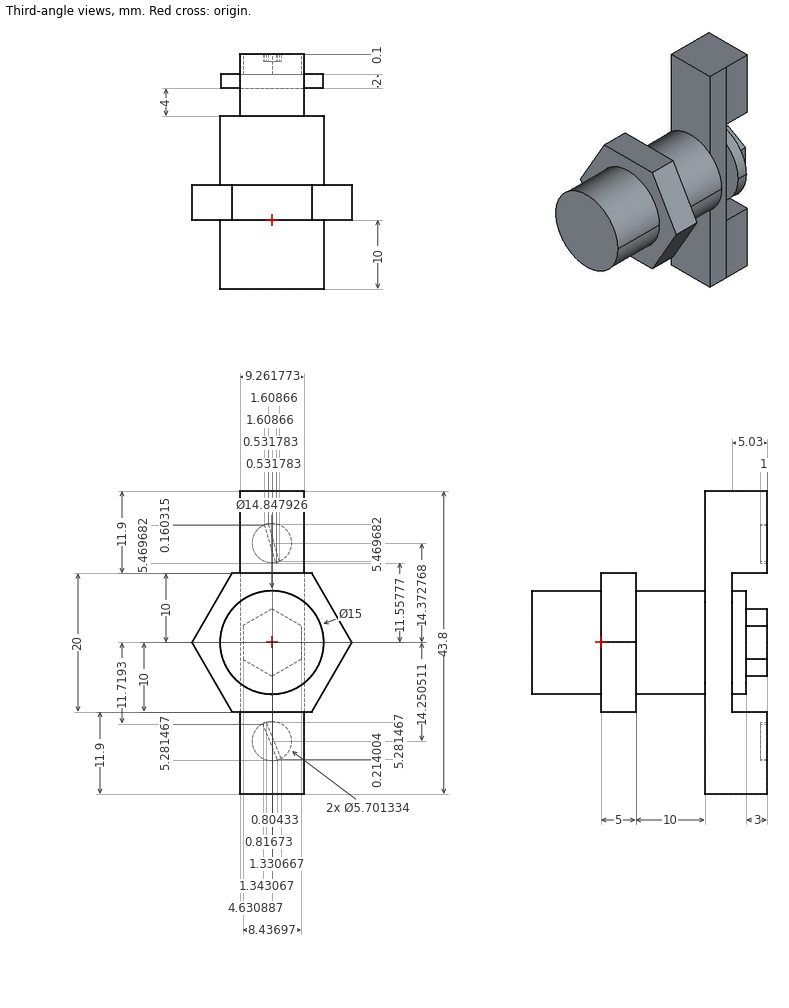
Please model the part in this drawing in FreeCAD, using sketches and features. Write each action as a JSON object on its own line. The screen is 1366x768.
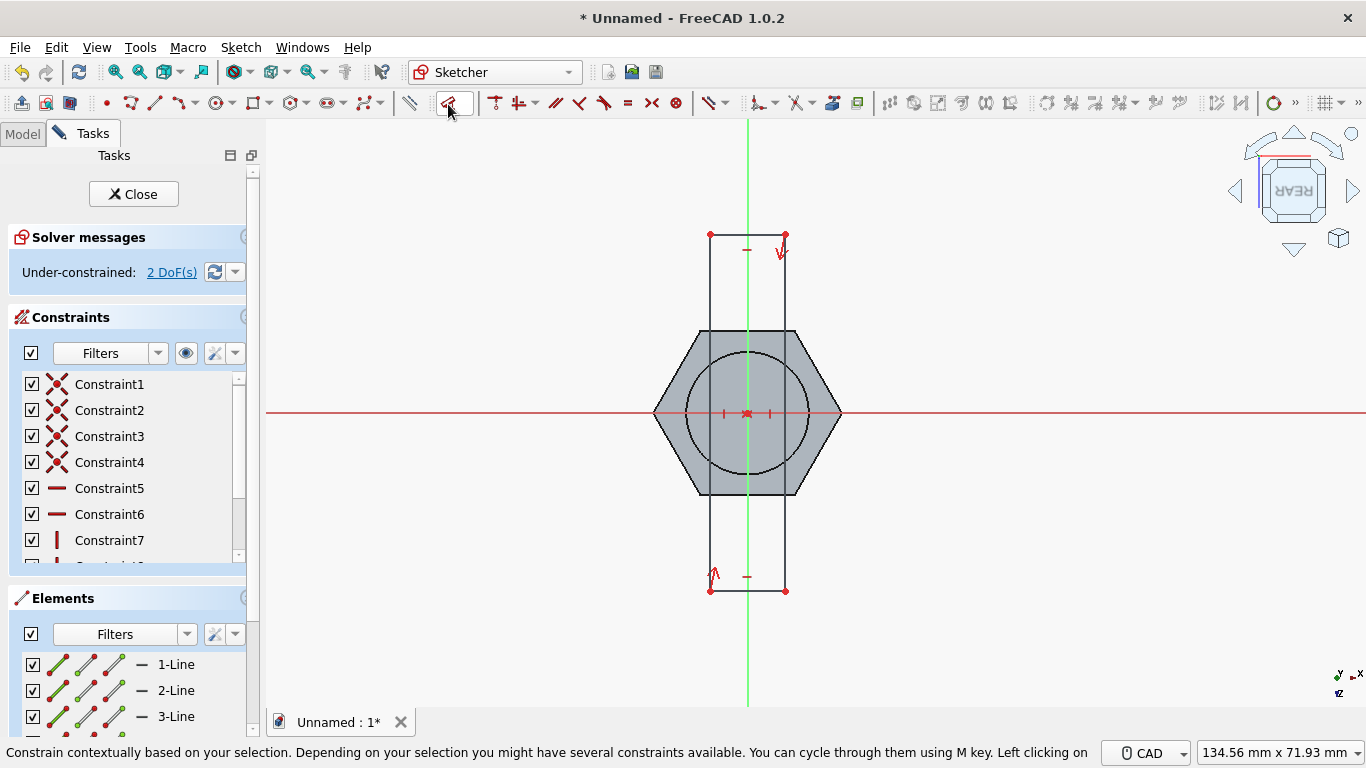
{"action": "left_click", "coordinate": [785, 485]}
{"action": "left_click", "coordinate": [819, 331]}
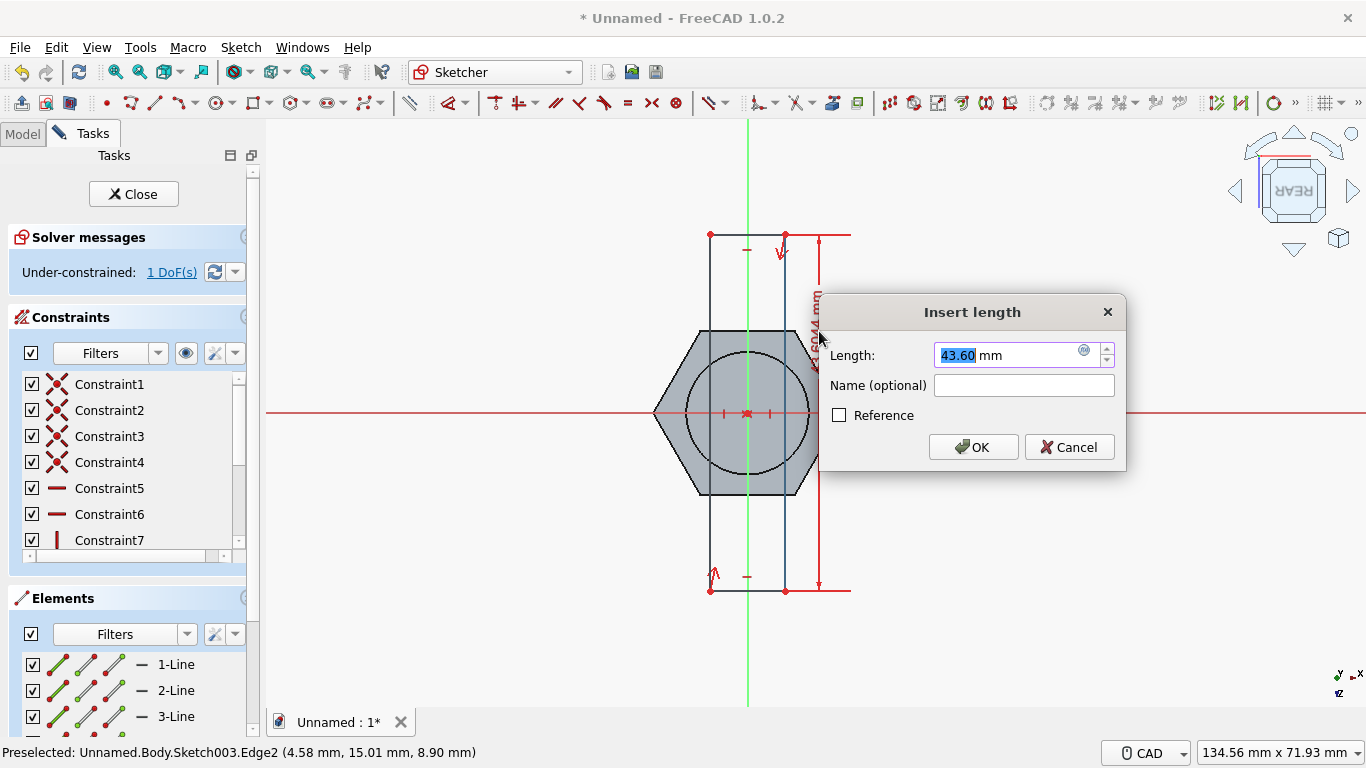
{"action": "type", "text": "43.8"}
{"action": "key", "text": "Return"}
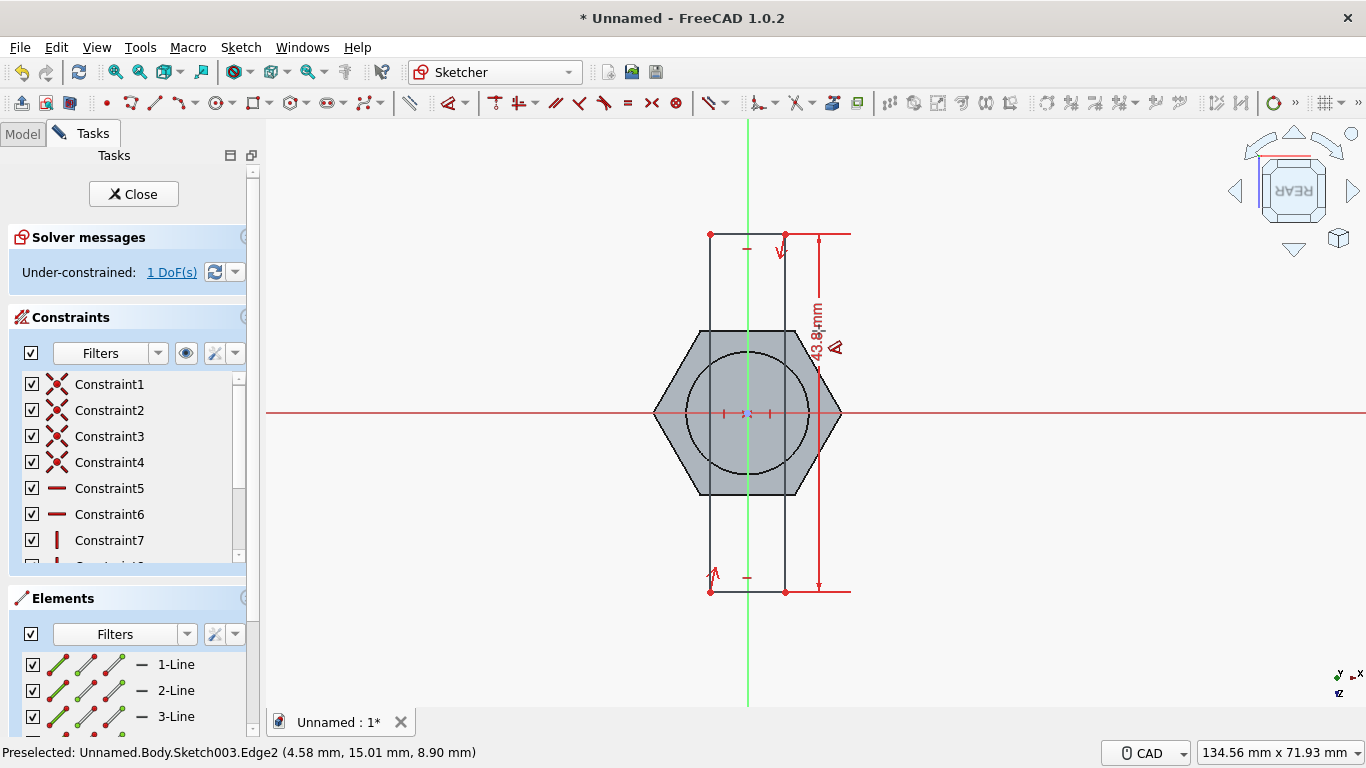
{"action": "left_click", "coordinate": [733, 592]}
{"action": "left_click", "coordinate": [730, 626]}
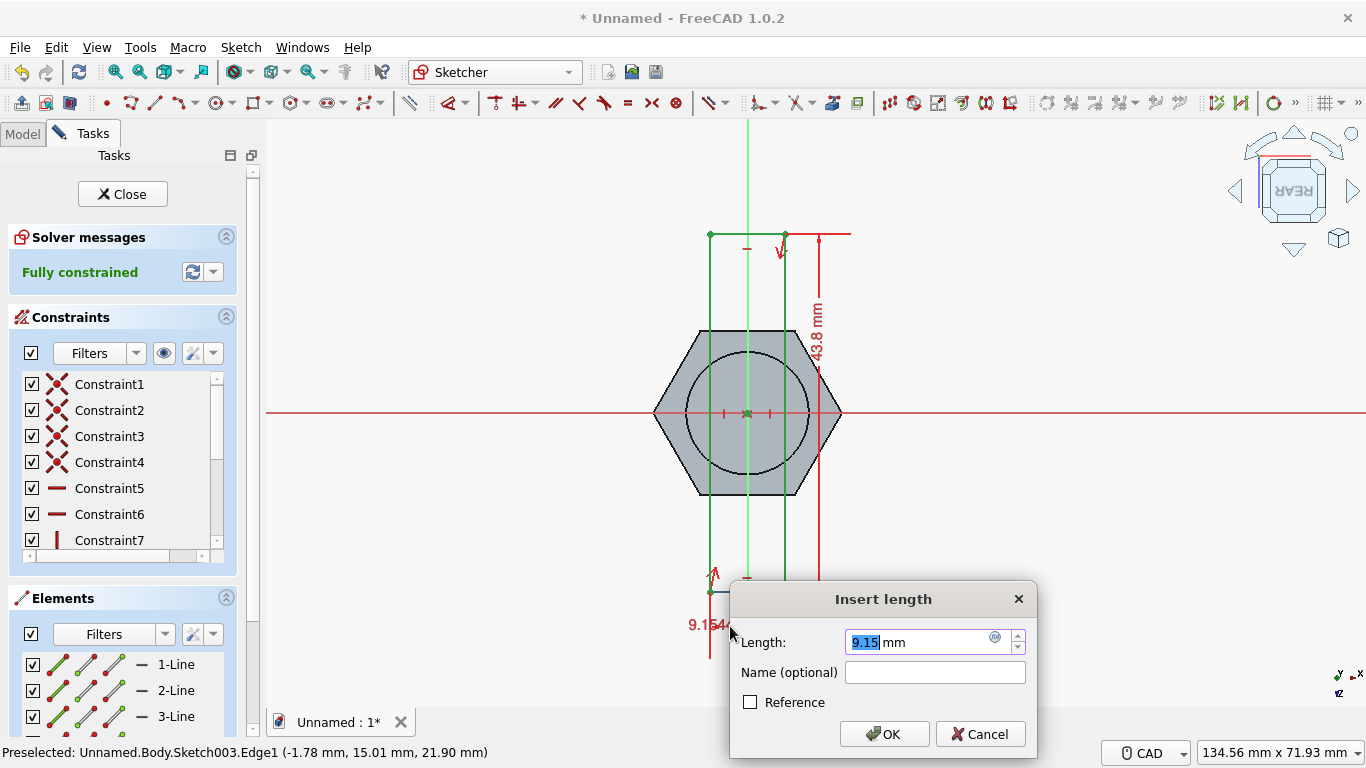
{"action": "type", "text": "9.261773"}
{"action": "key", "text": "Return"}
{"action": "key", "text": "Escape"}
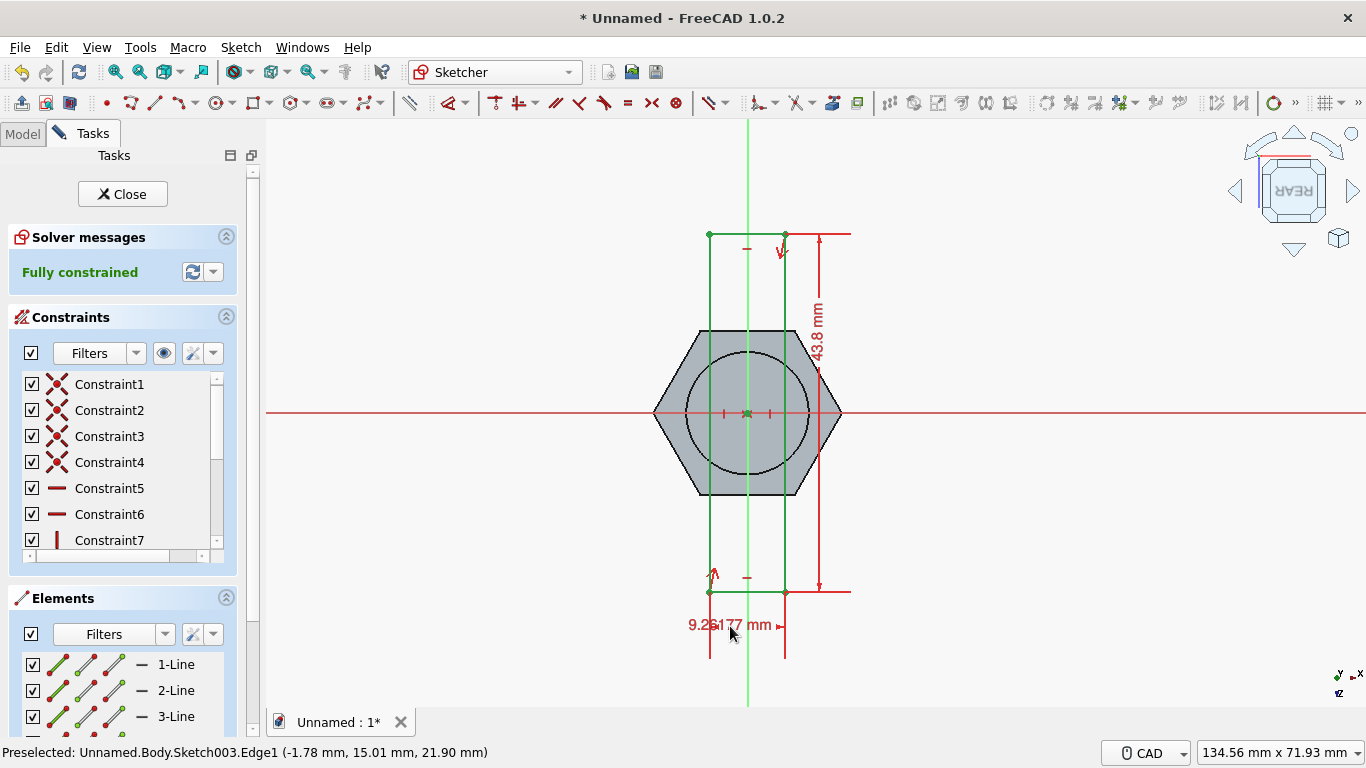
{"action": "left_click", "coordinate": [123, 194]}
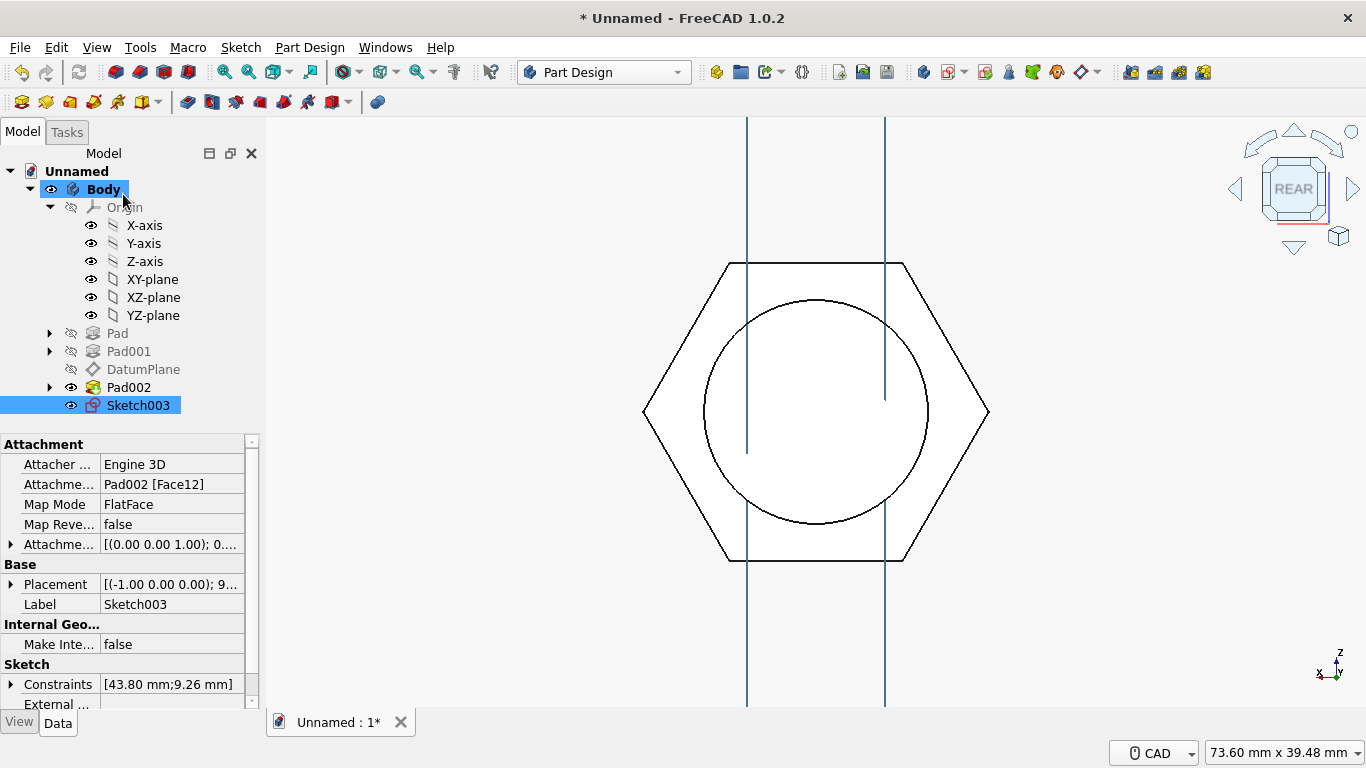
{"action": "left_click", "coordinate": [22, 102]}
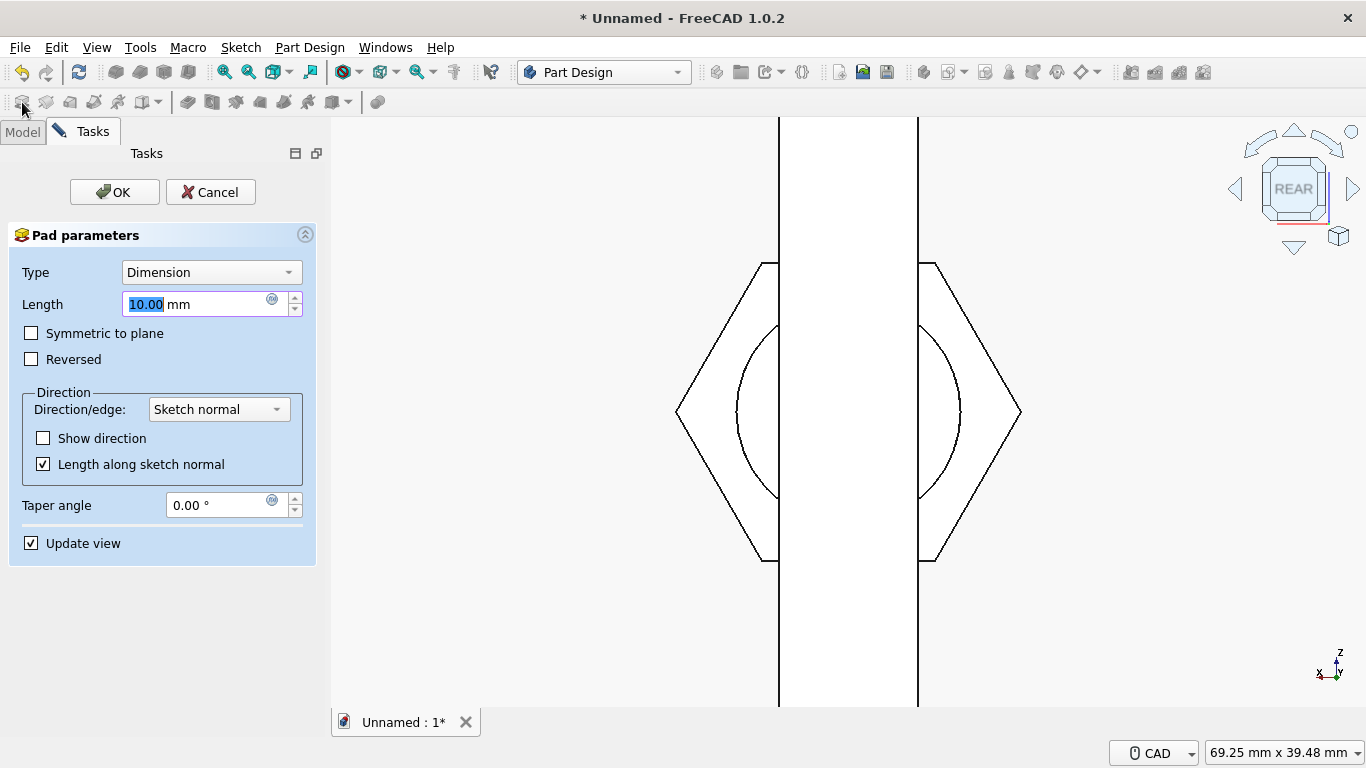
{"action": "type", "text": "4"}
{"action": "key", "text": "Tab"}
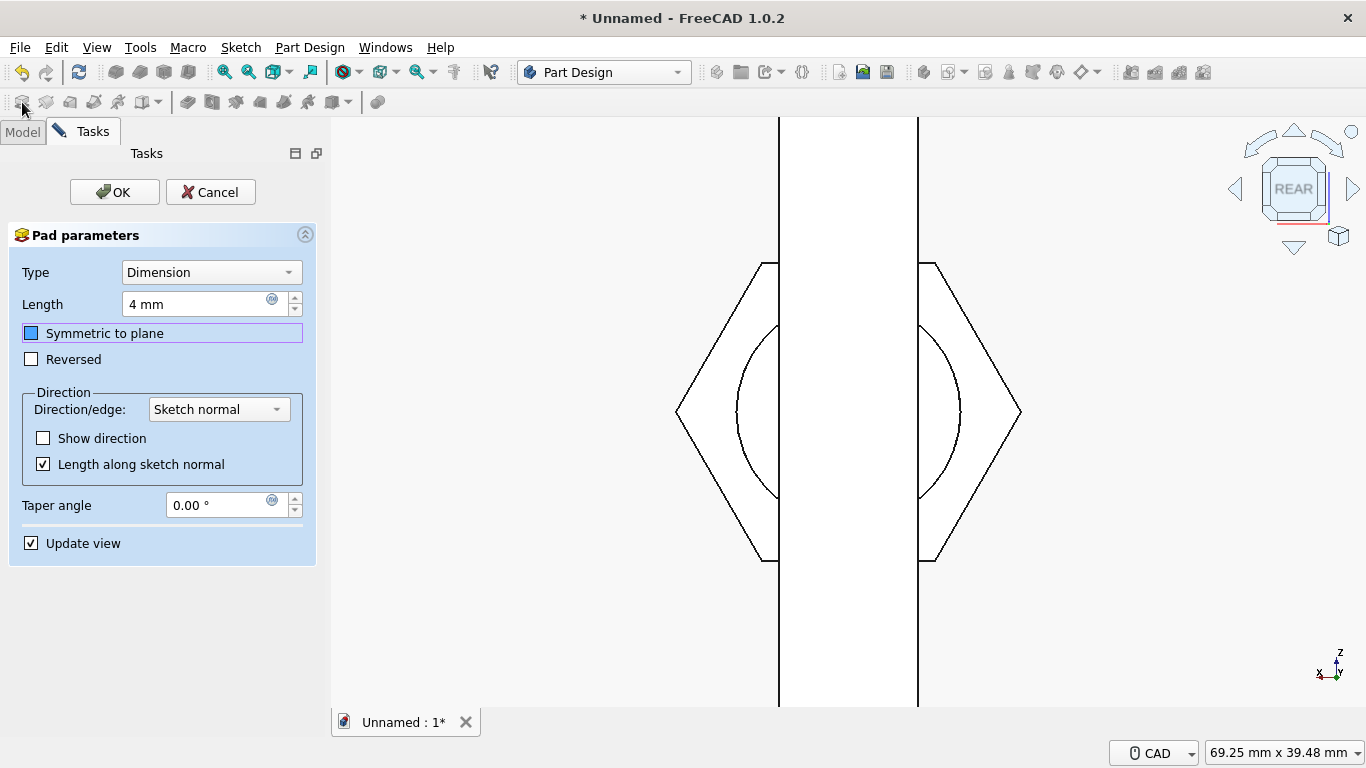
{"action": "left_click", "coordinate": [115, 192]}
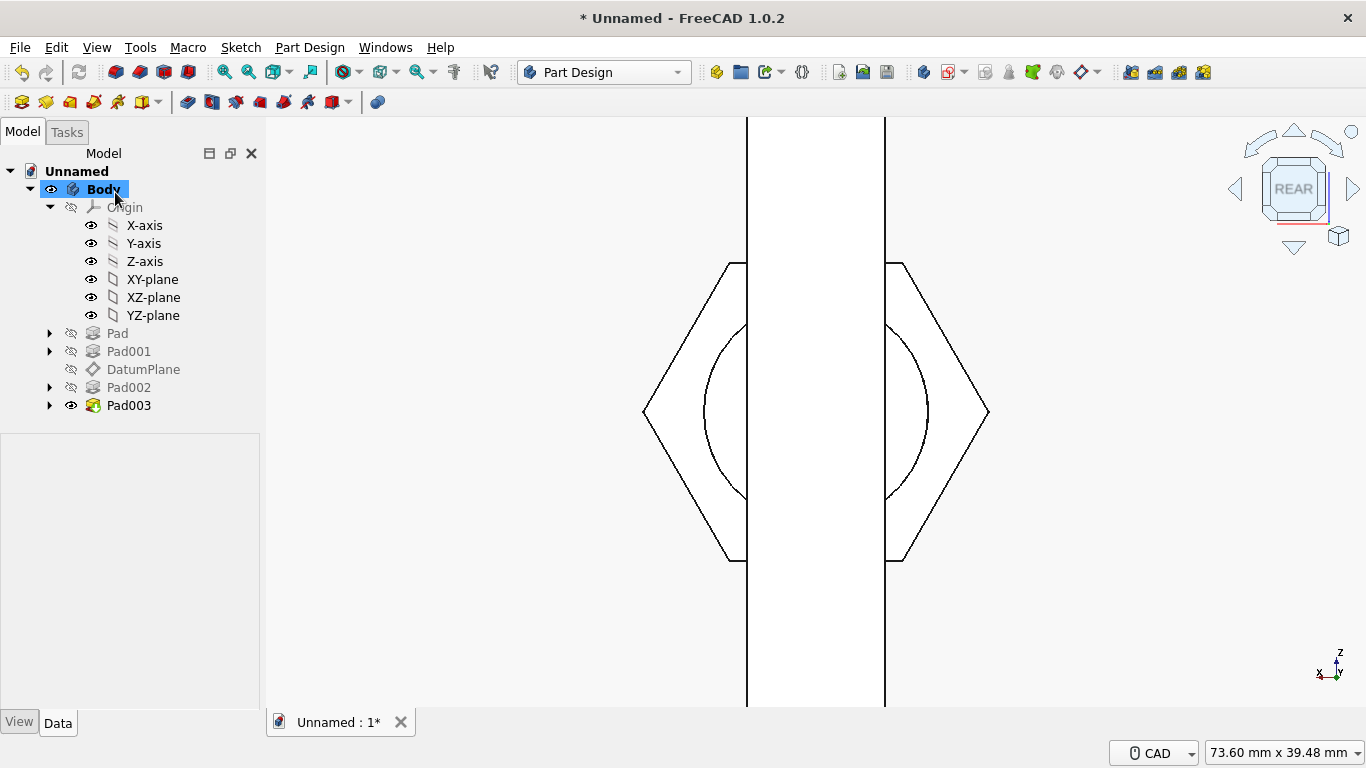
{"action": "left_click", "coordinate": [226, 72]}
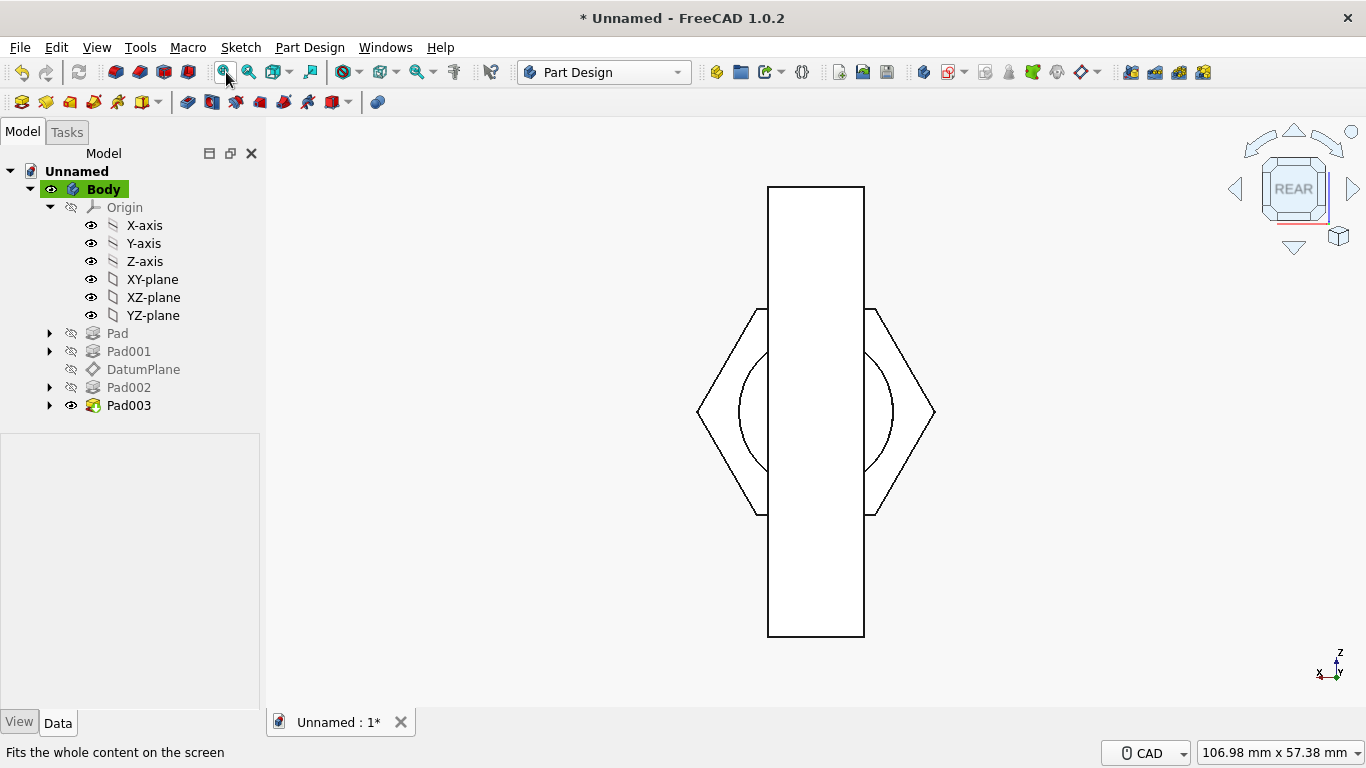
{"action": "left_click", "coordinate": [816, 540]}